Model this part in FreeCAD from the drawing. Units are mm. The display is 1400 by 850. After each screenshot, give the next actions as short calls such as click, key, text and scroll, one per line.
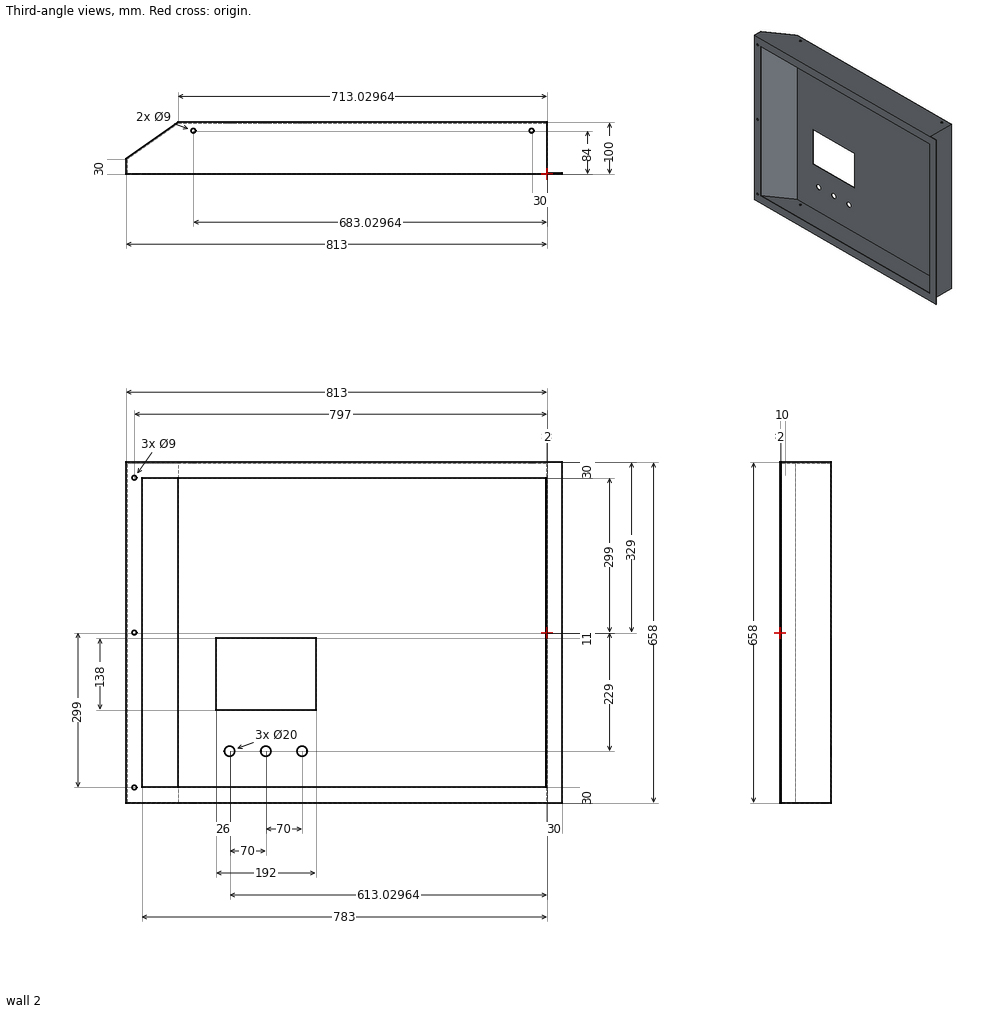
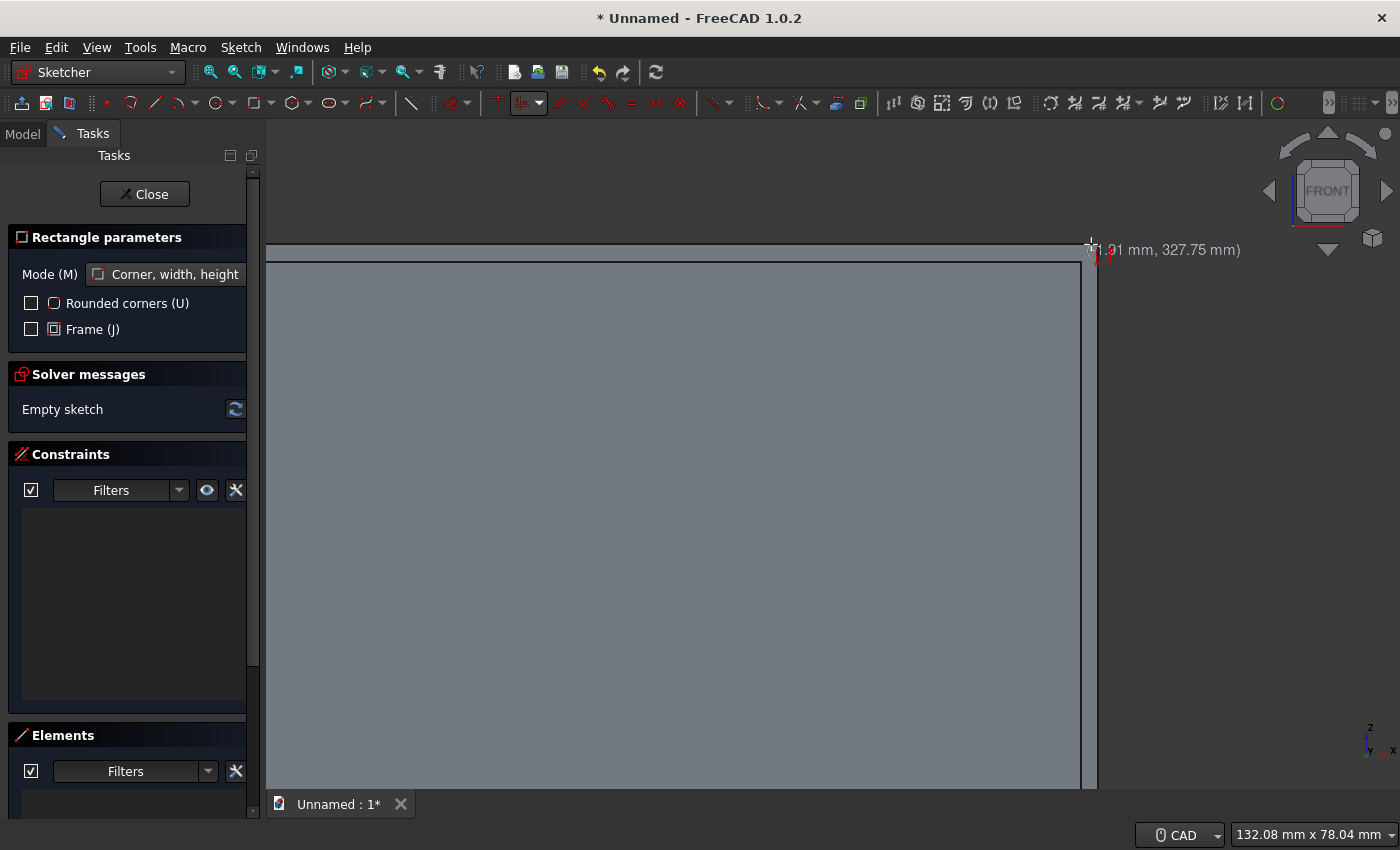
click(1081, 244)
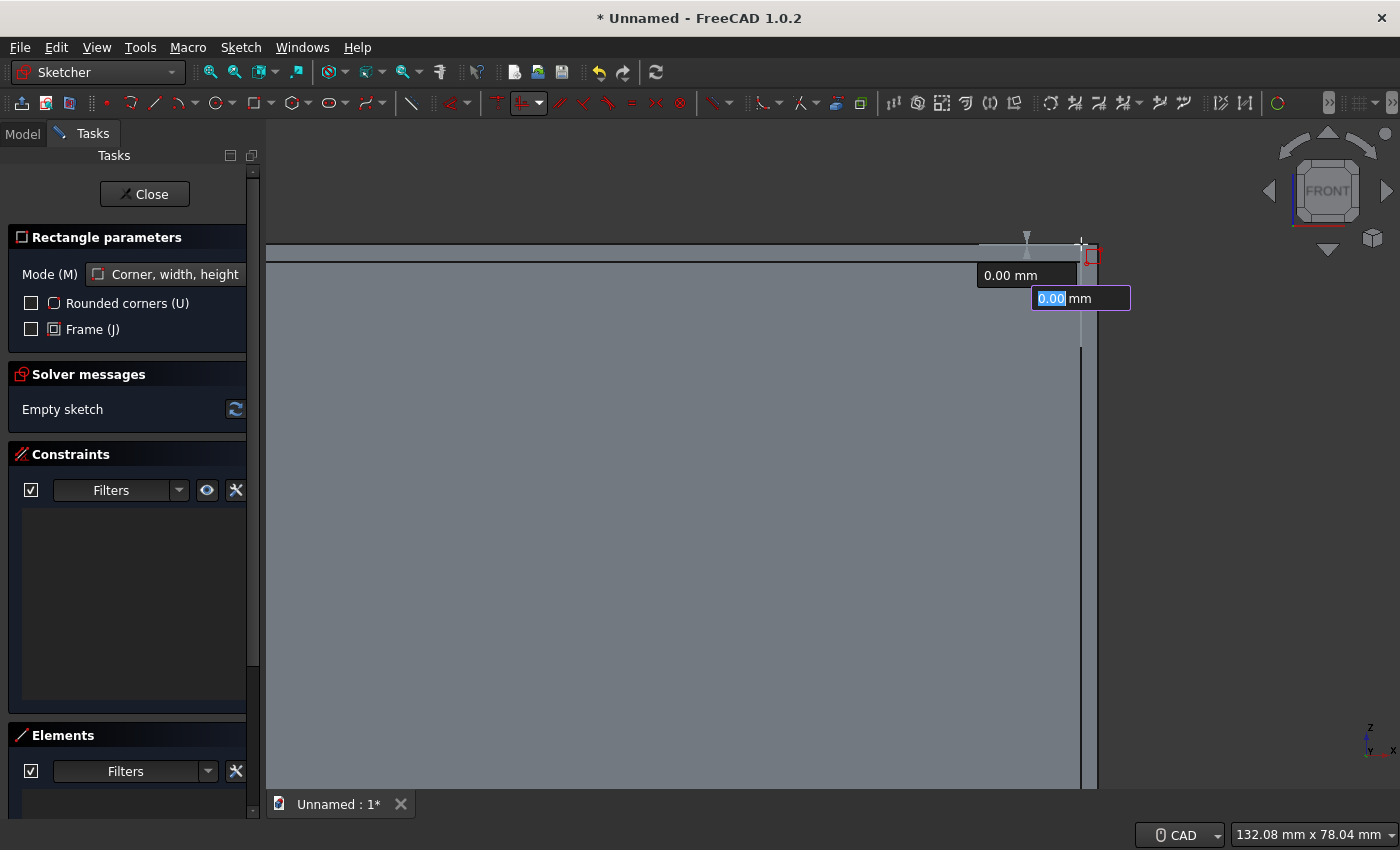
scroll(729, 244, down, 13)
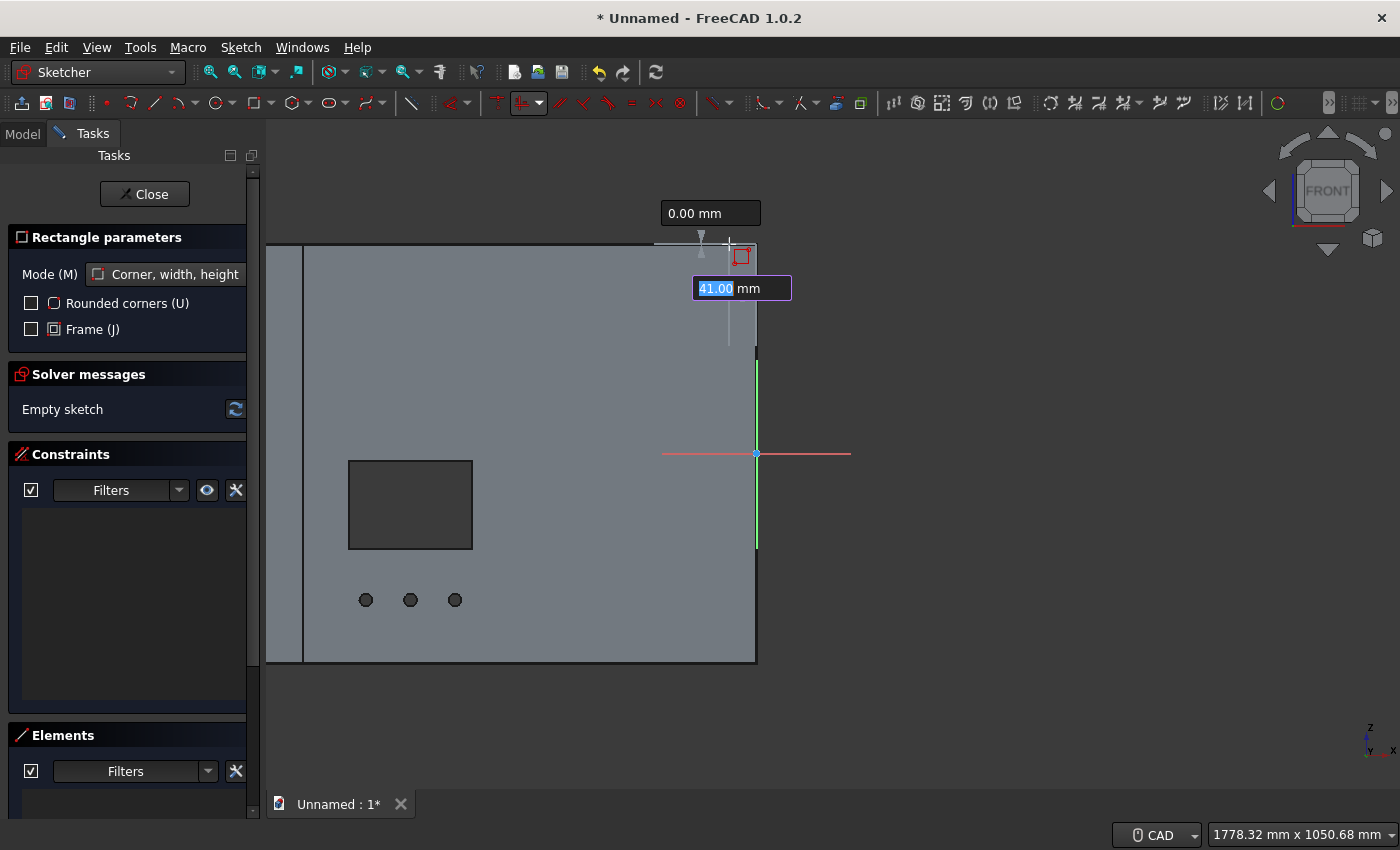
click(775, 664)
key(Escape)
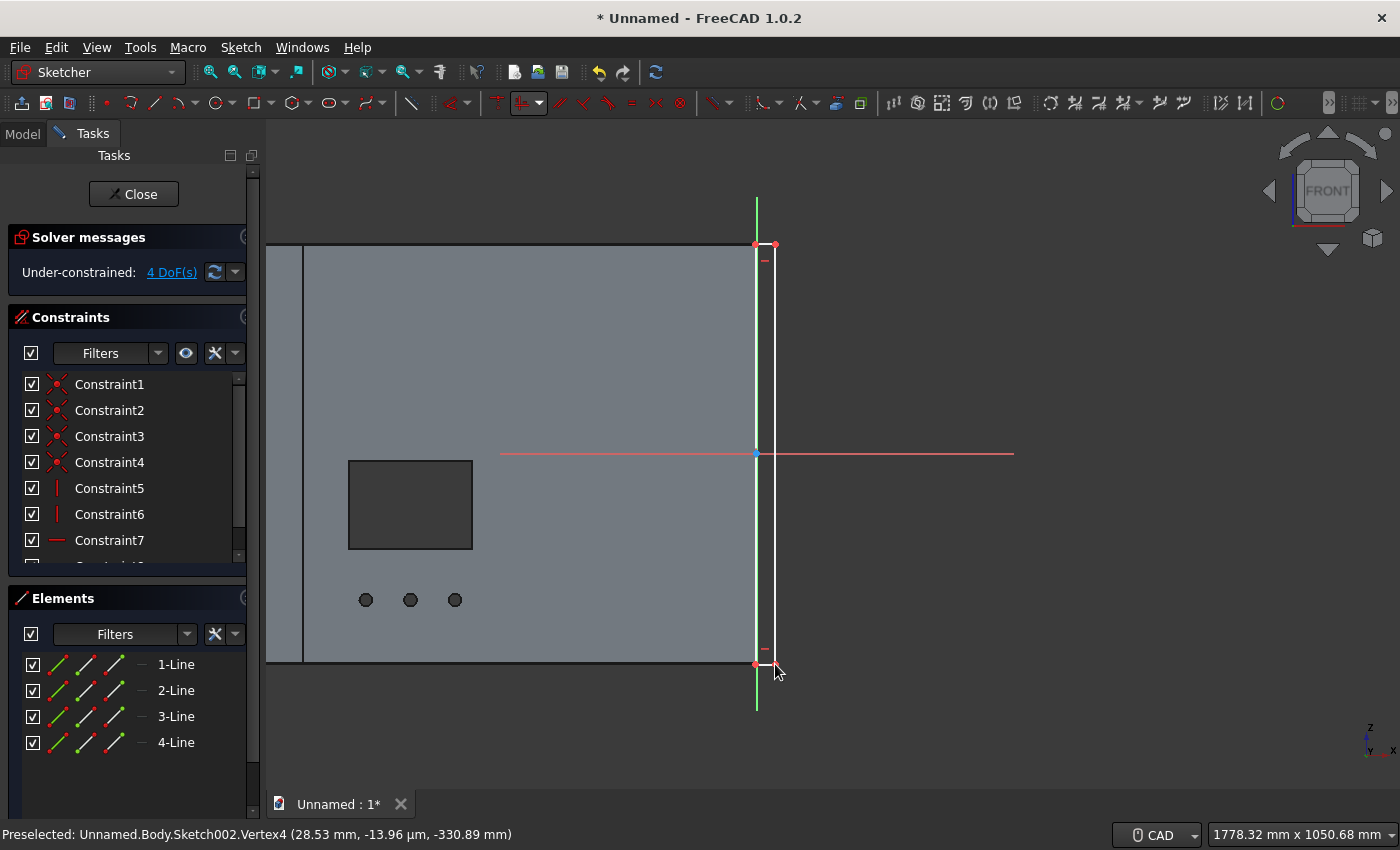
key(d)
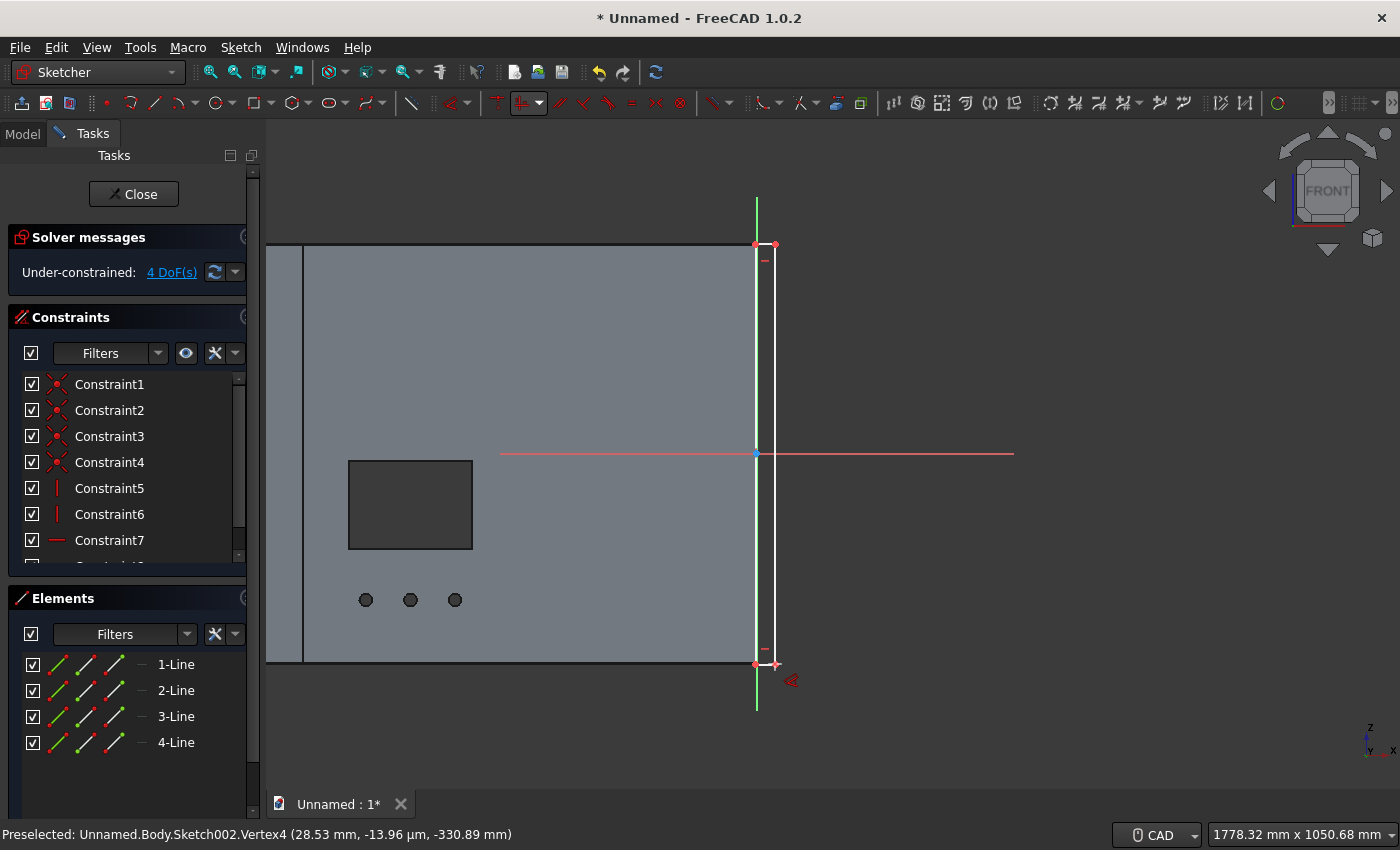
scroll(765, 665, up, 4)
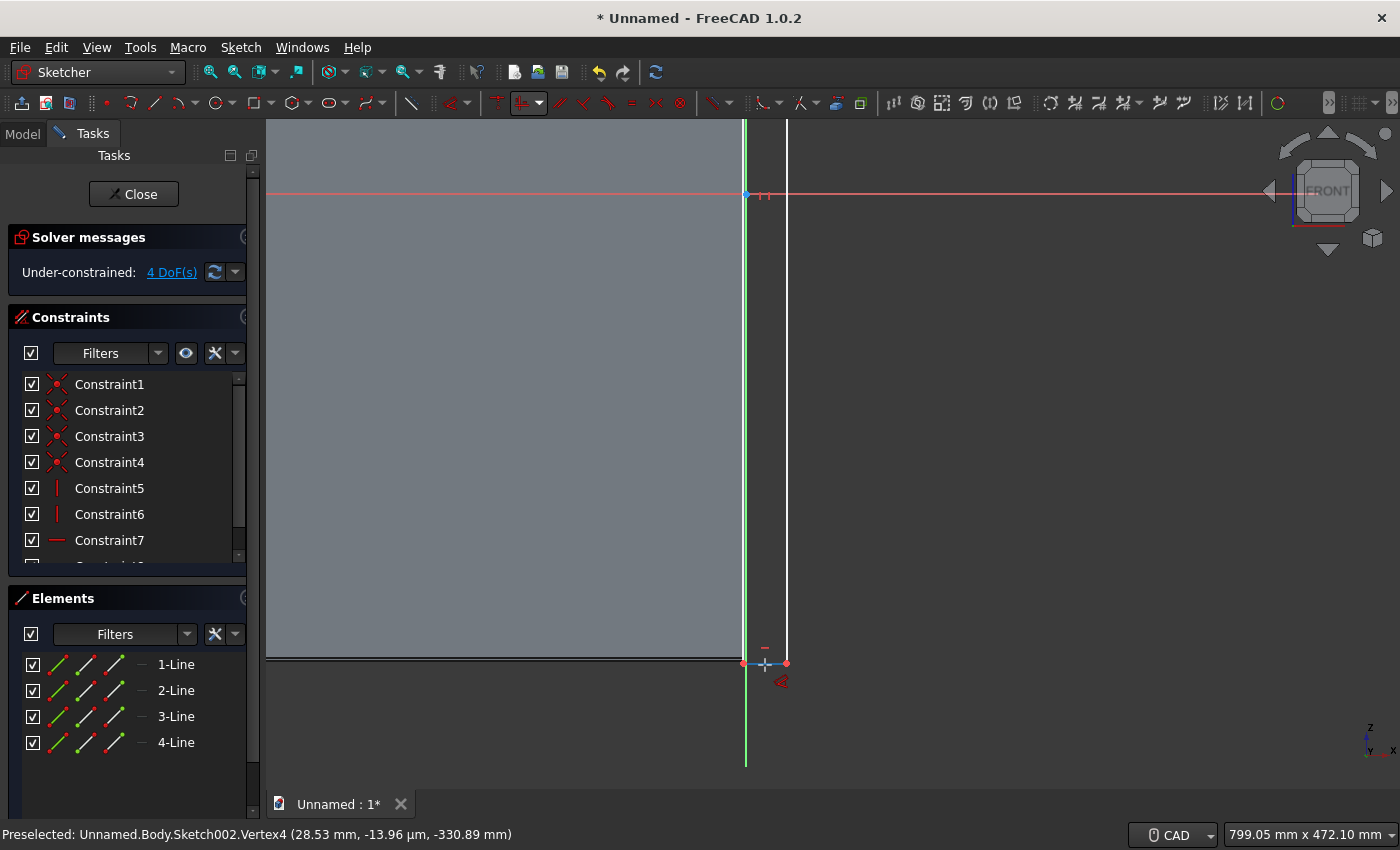
click(765, 664)
click(765, 698)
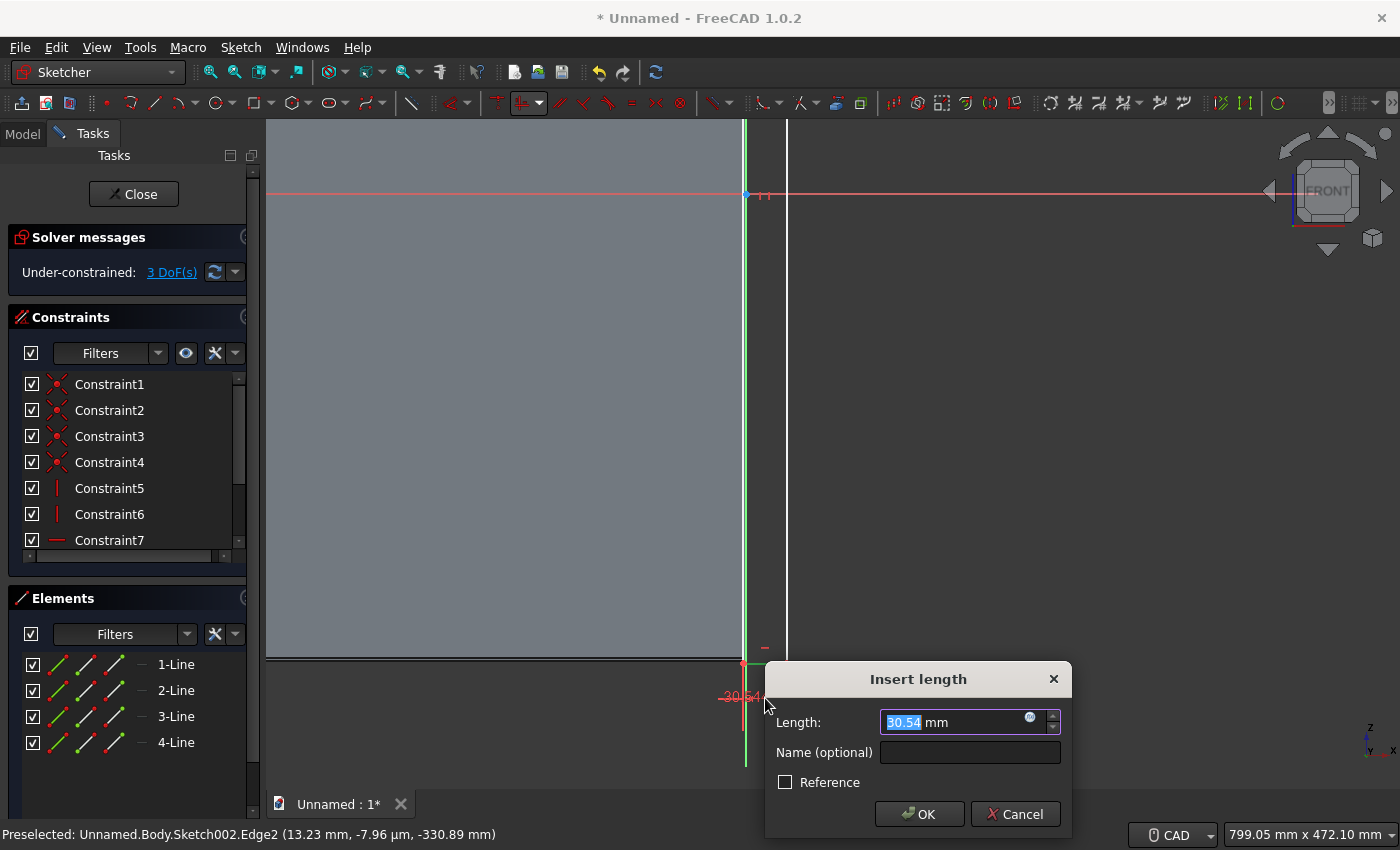
text(30)
key(Return)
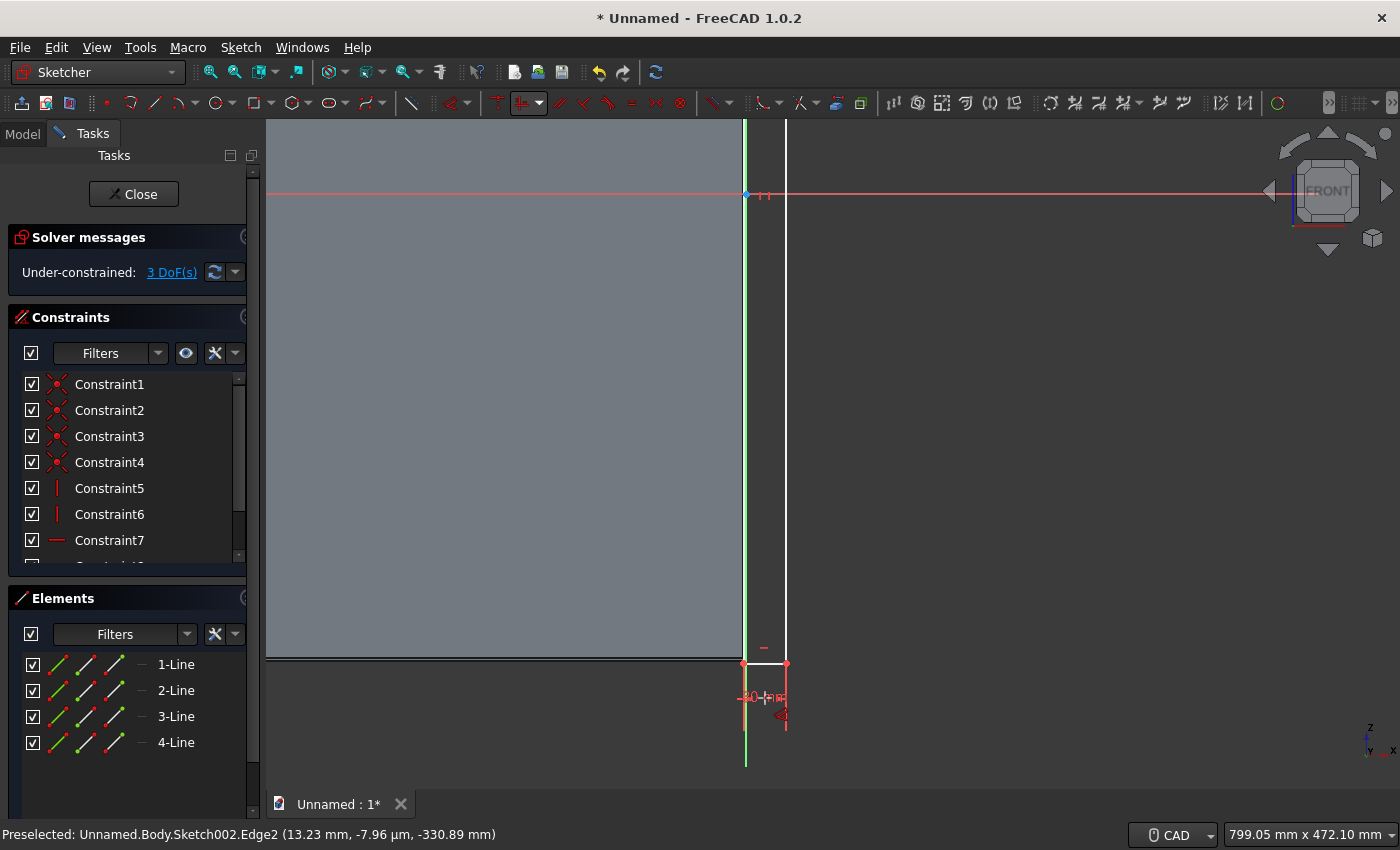
scroll(764, 666, down, 4)